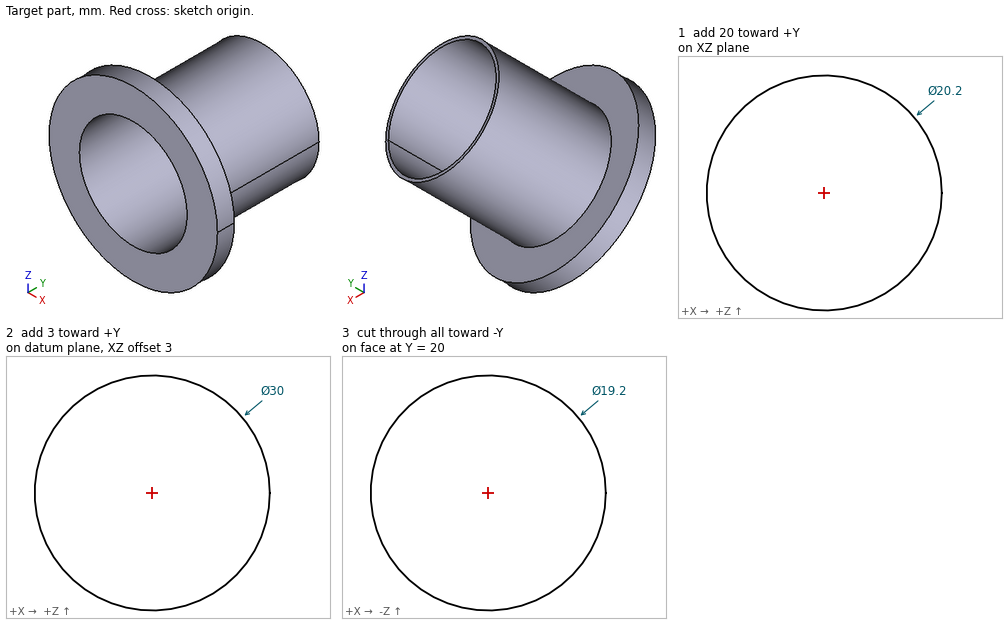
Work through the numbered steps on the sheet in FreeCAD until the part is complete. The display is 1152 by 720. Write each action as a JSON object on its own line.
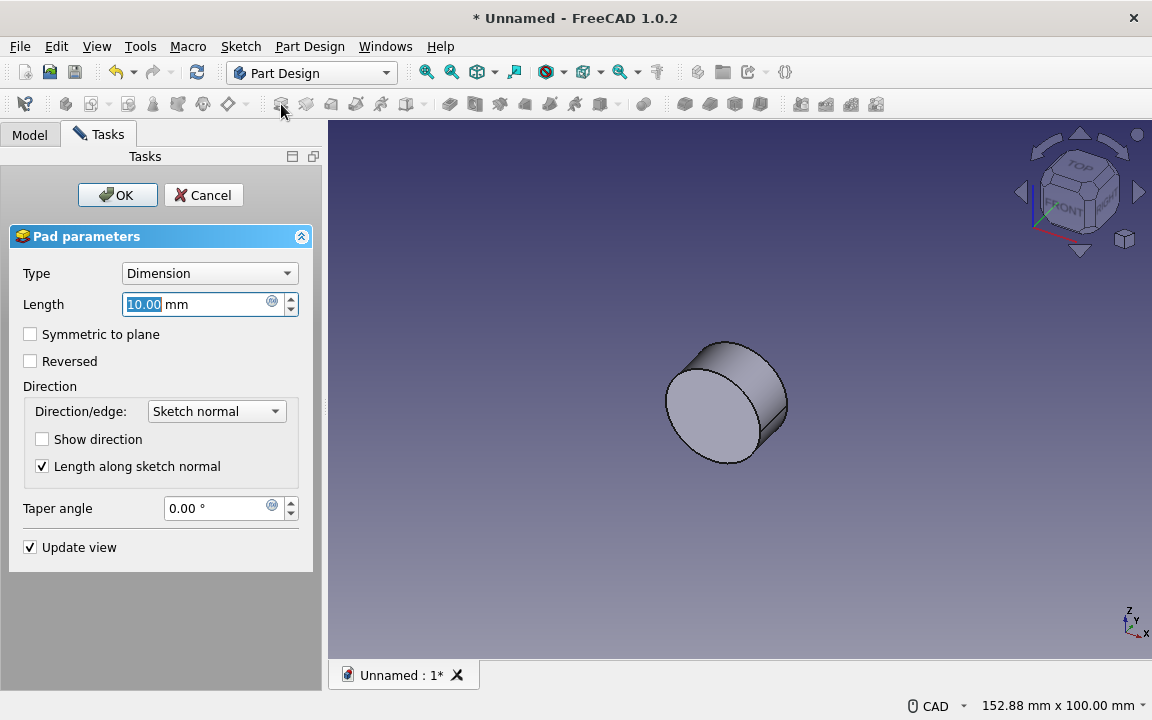
{"action": "type", "text": "20"}
{"action": "key", "text": "Tab"}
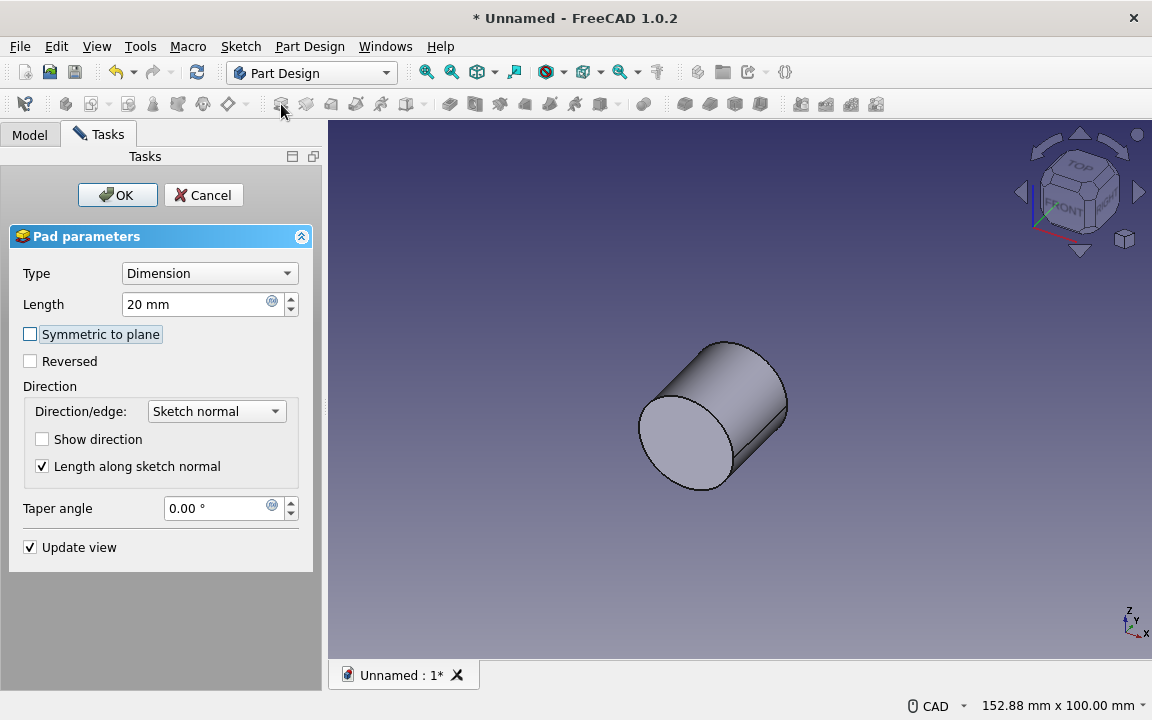
{"action": "left_click", "coordinate": [31, 361]}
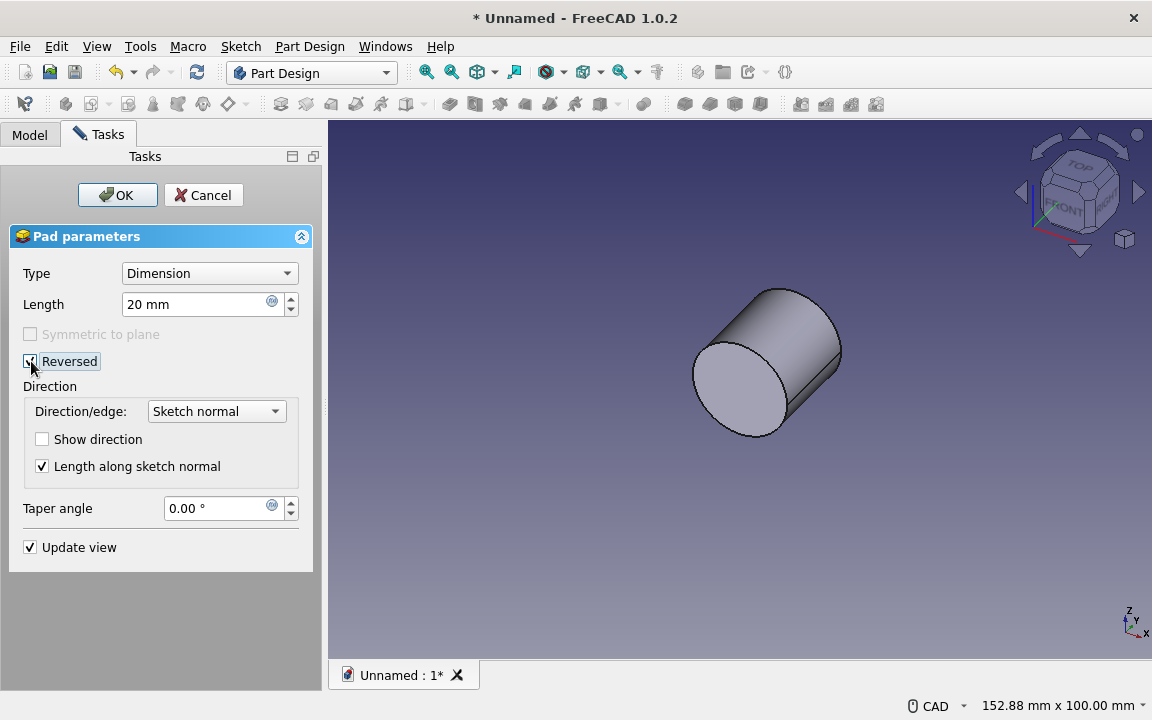
{"action": "left_click", "coordinate": [118, 195]}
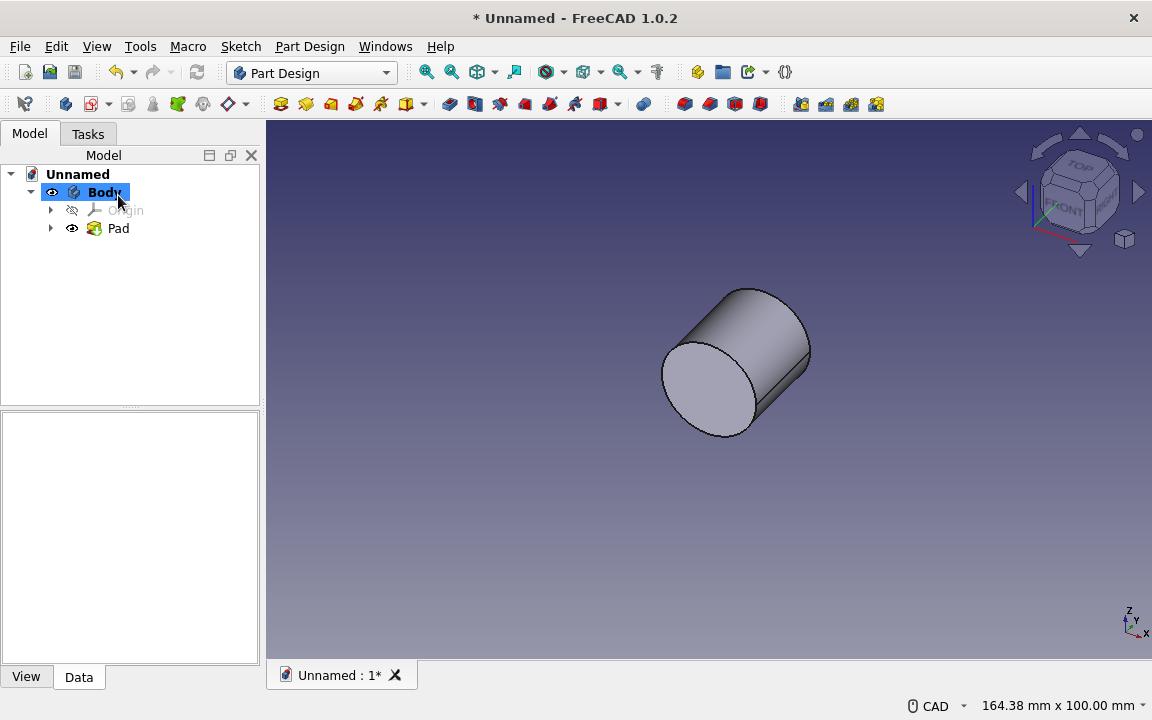
{"action": "key", "text": "v f"}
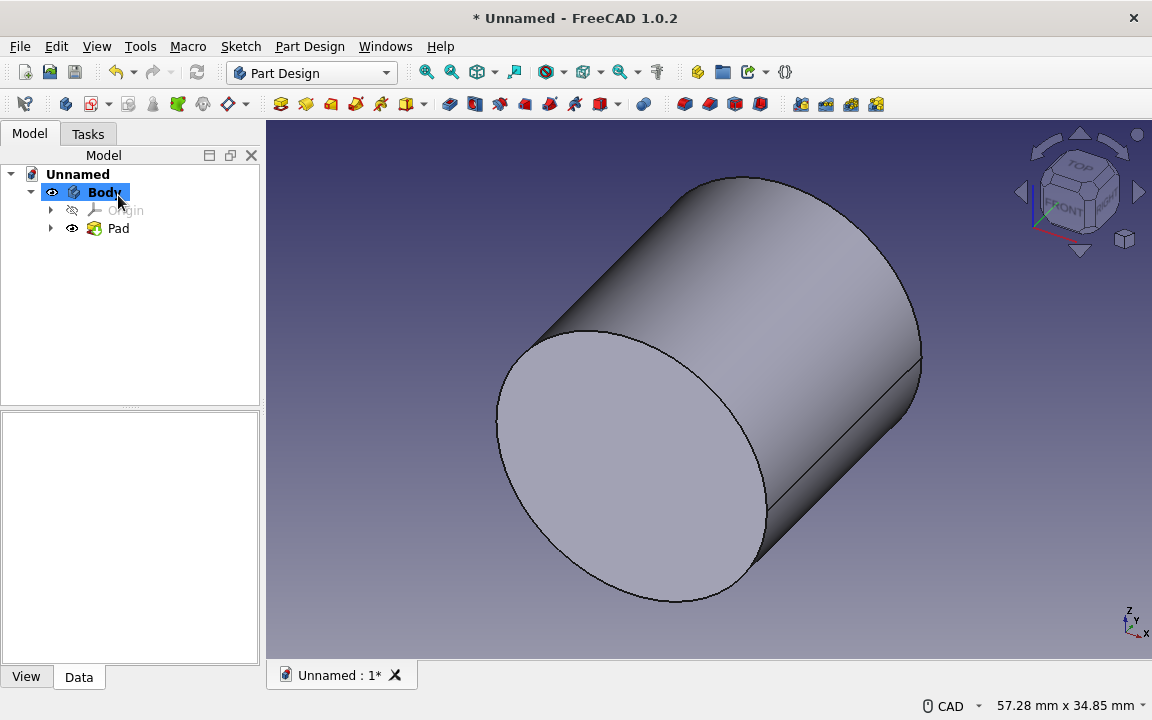
{"action": "left_click", "coordinate": [51, 210]}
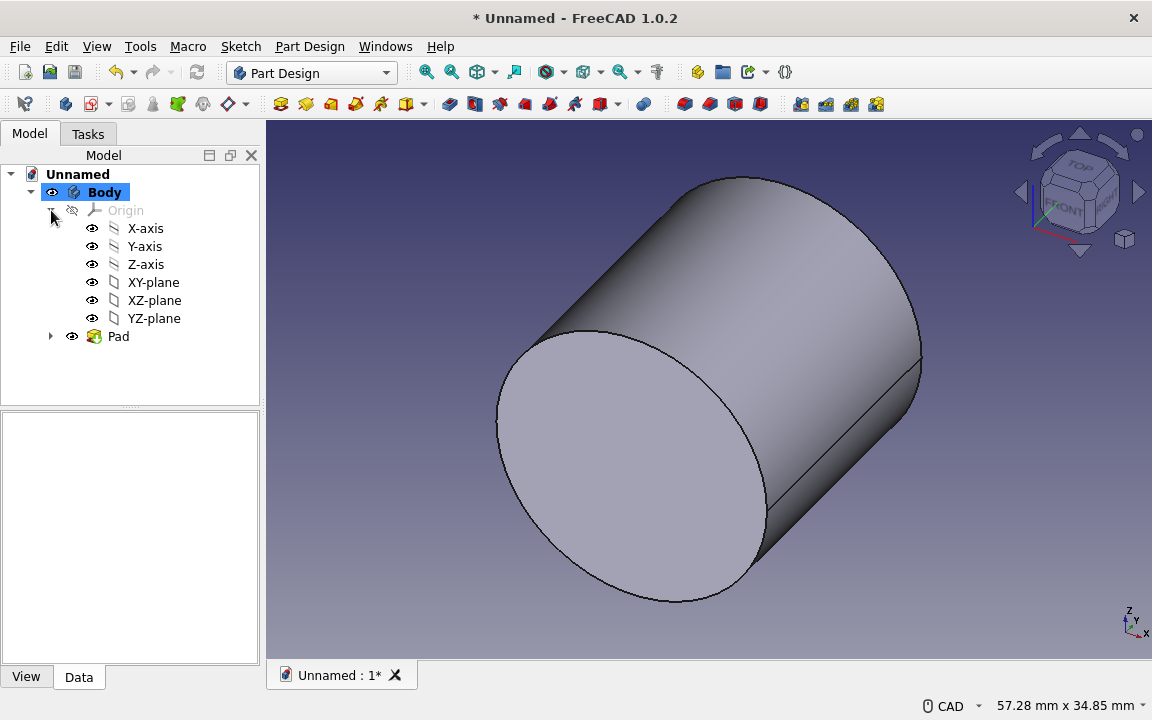
{"action": "left_click", "coordinate": [137, 300]}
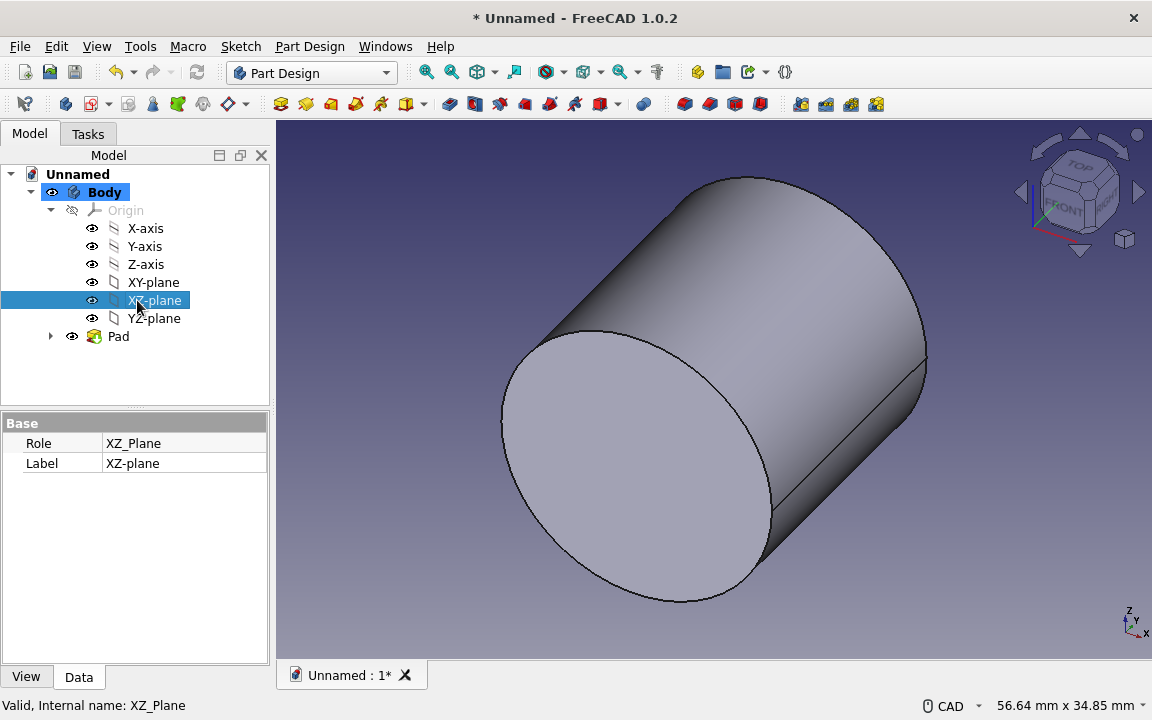
{"action": "left_click", "coordinate": [228, 104]}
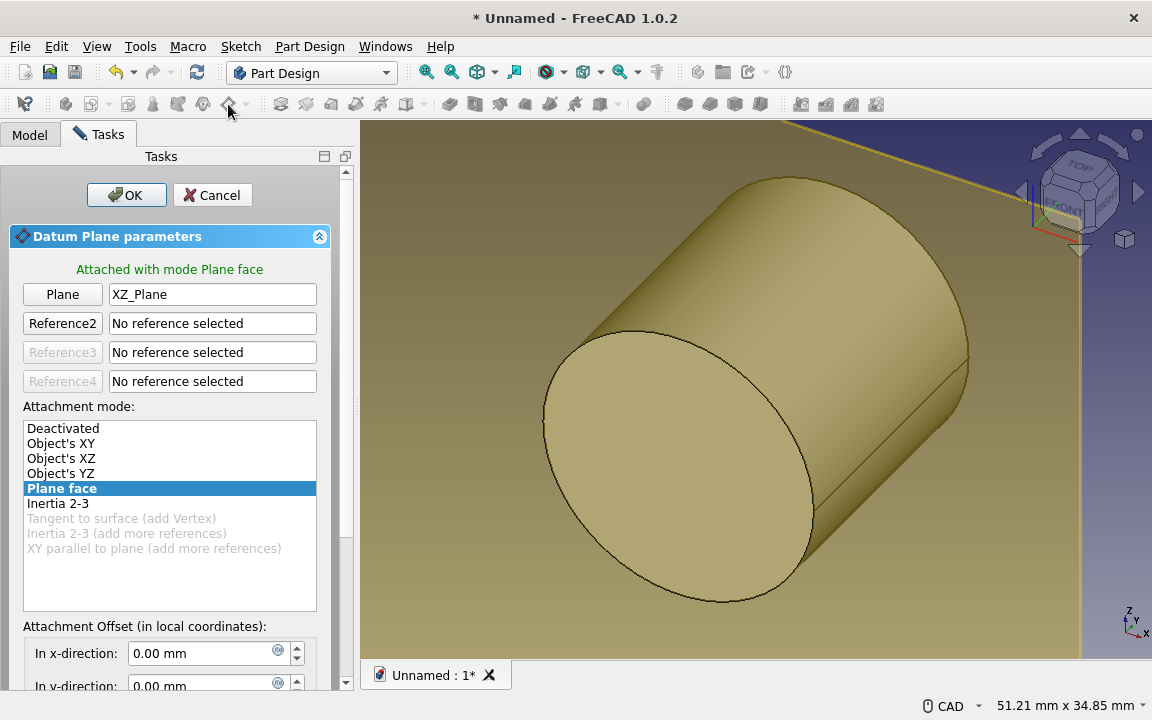
{"action": "scroll", "coordinate": [346, 428], "scroll_direction": "down", "scroll_amount": 2}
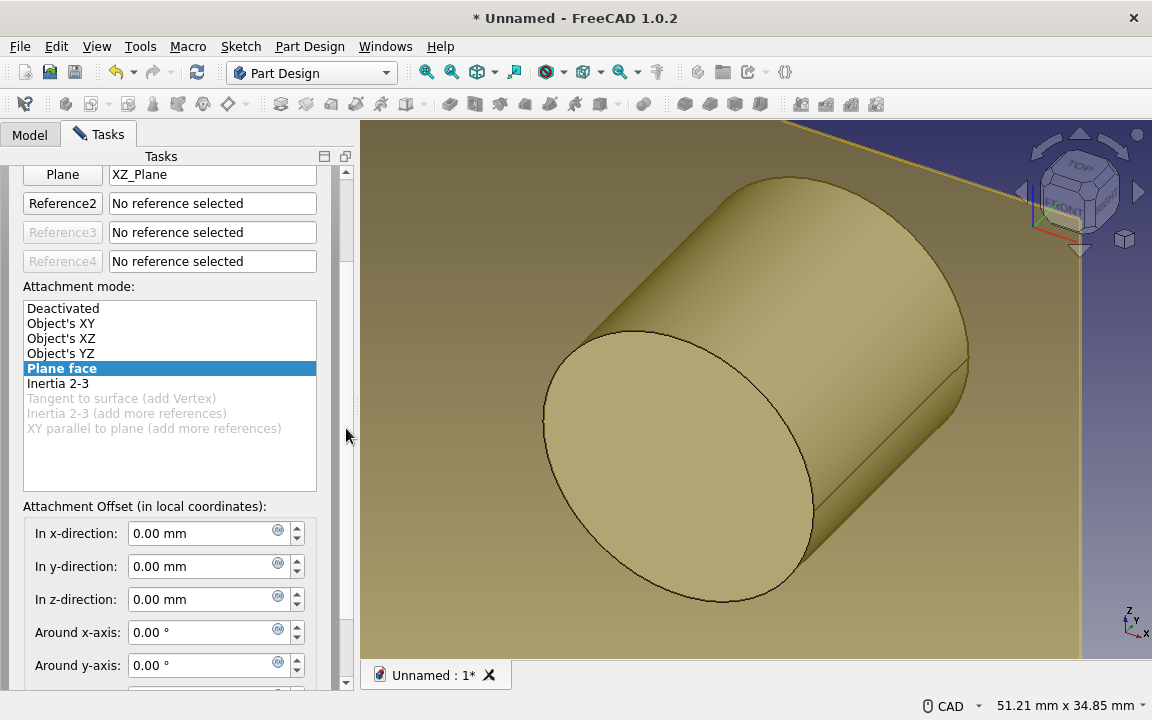
{"action": "triple_click", "coordinate": [210, 600]}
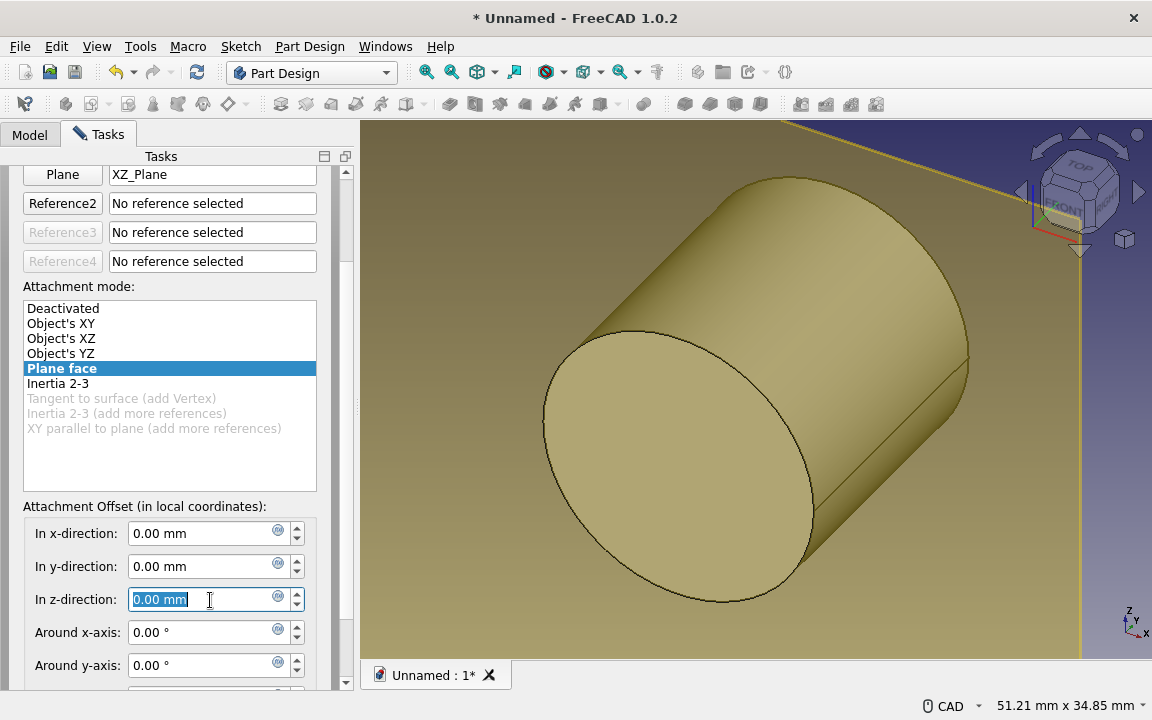
{"action": "type", "text": "3"}
{"action": "key", "text": "Tab"}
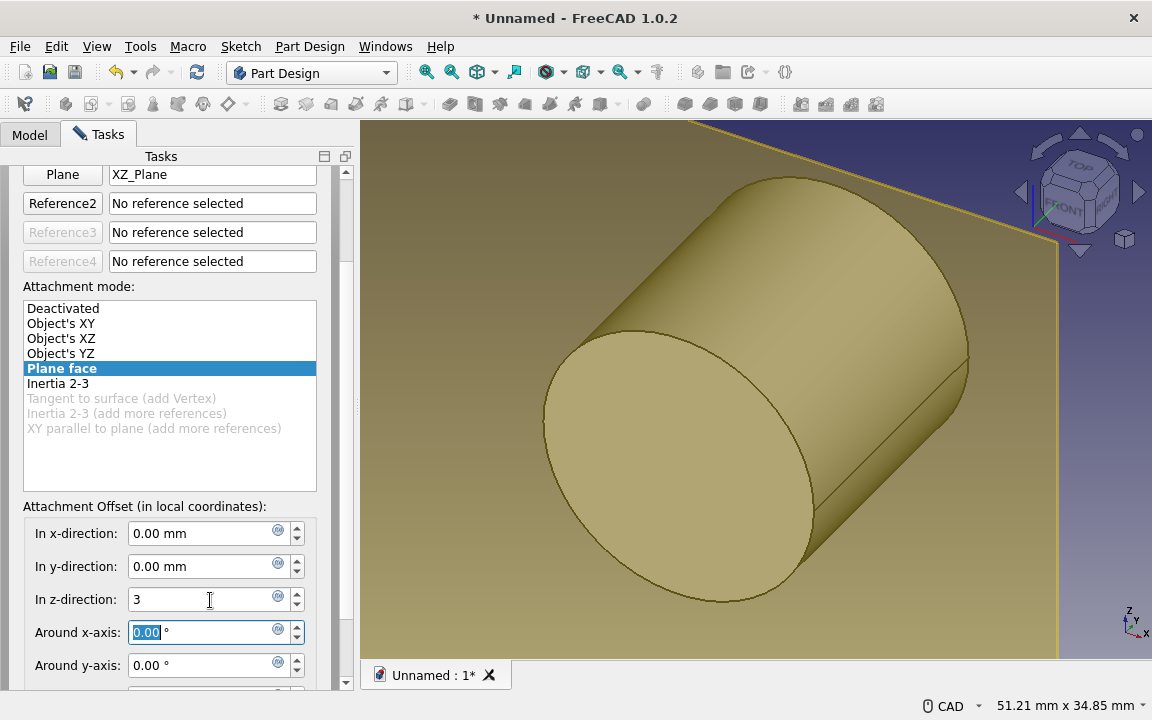
{"action": "scroll", "coordinate": [346, 428], "scroll_direction": "up", "scroll_amount": 3}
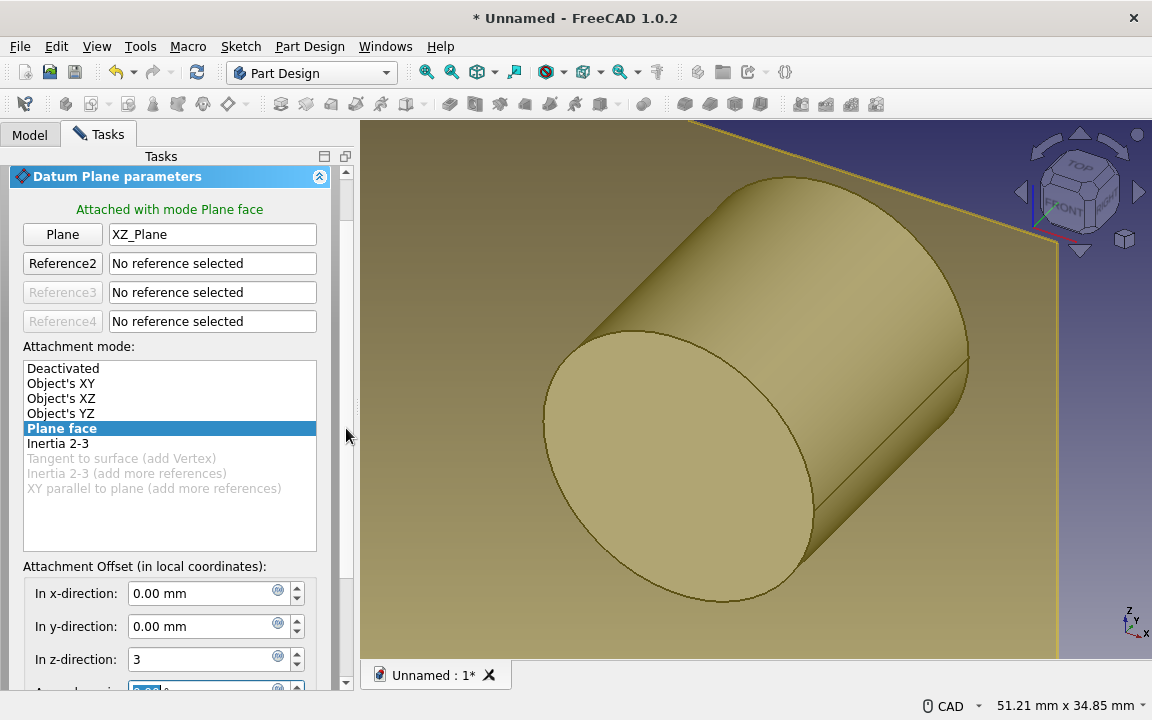
{"action": "left_click", "coordinate": [127, 195]}